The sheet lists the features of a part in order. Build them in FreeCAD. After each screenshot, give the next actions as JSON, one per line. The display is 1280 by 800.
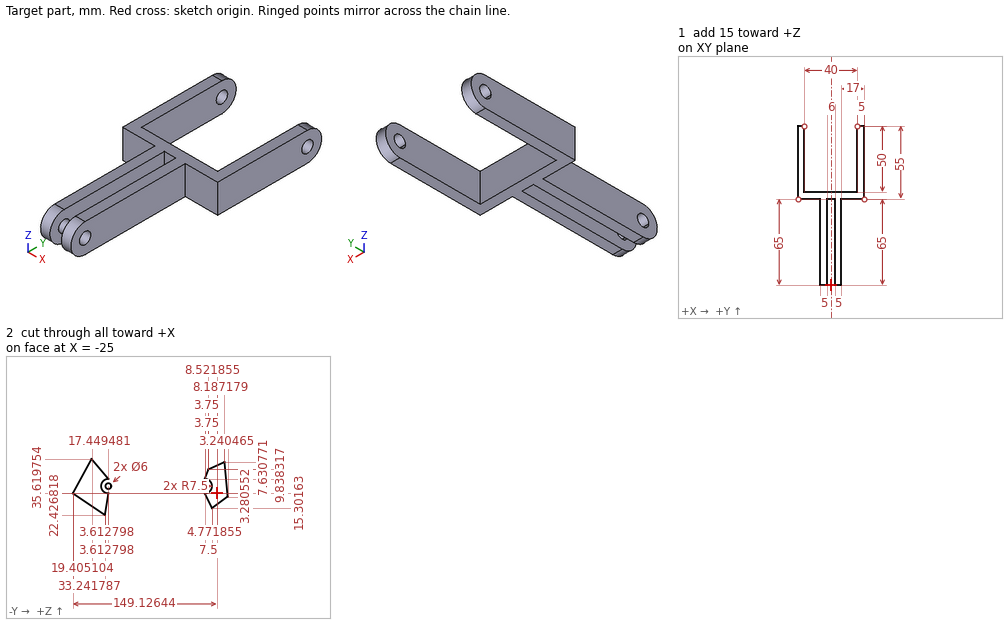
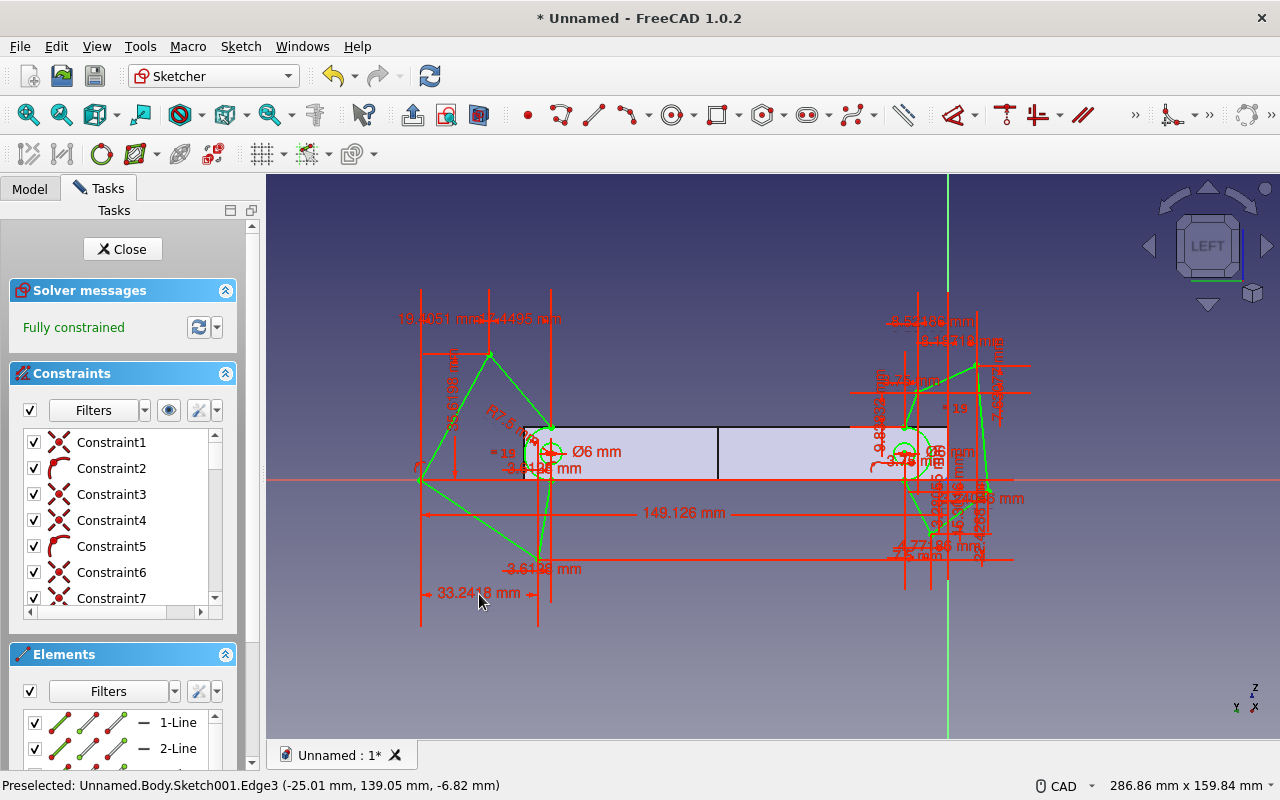
{"action": "left_click", "coordinate": [123, 249]}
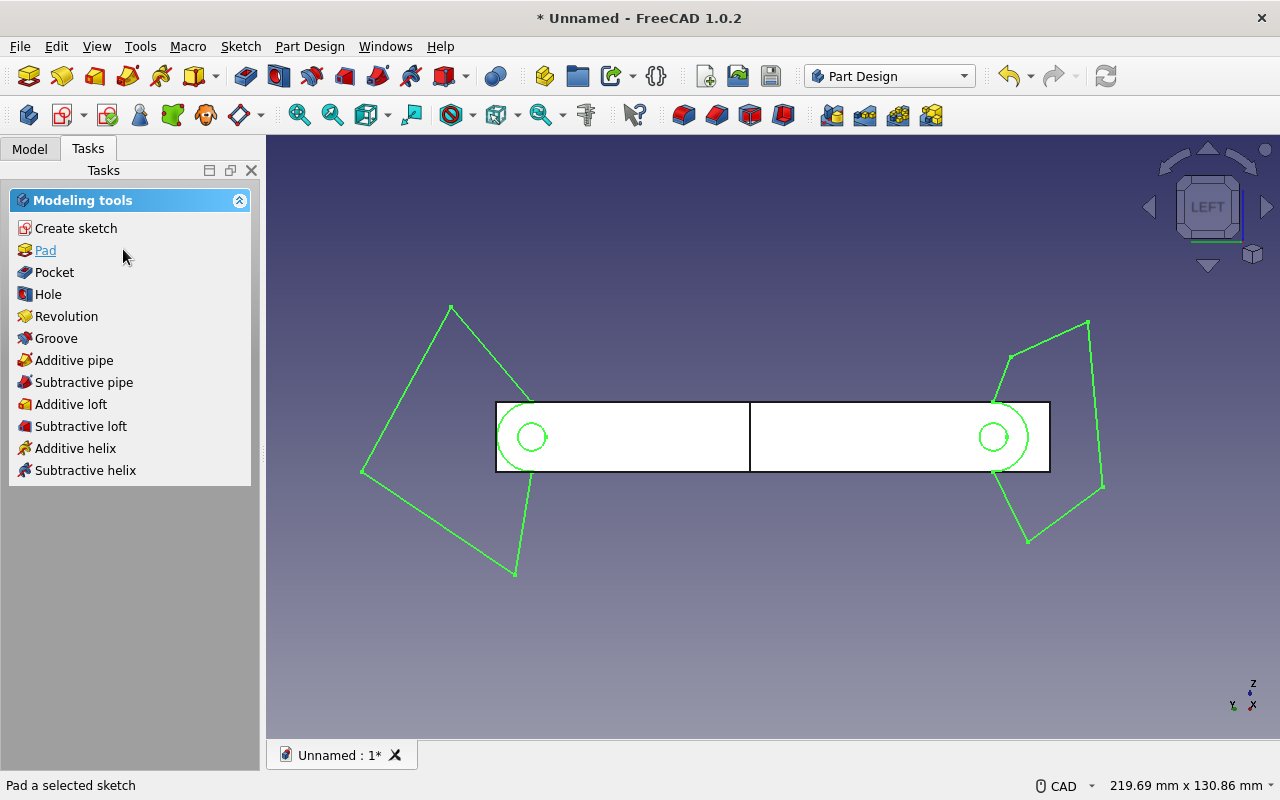
{"action": "left_click", "coordinate": [246, 76]}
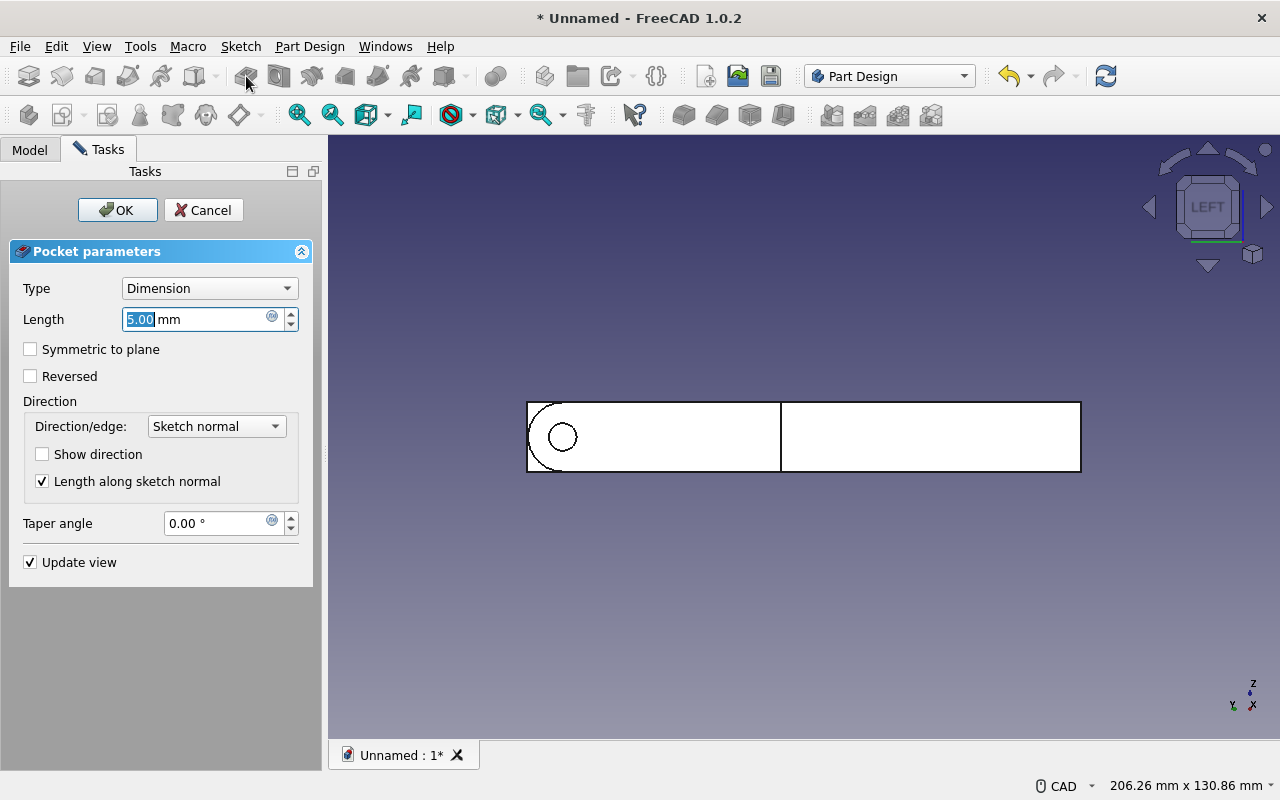
{"action": "left_click", "coordinate": [210, 288]}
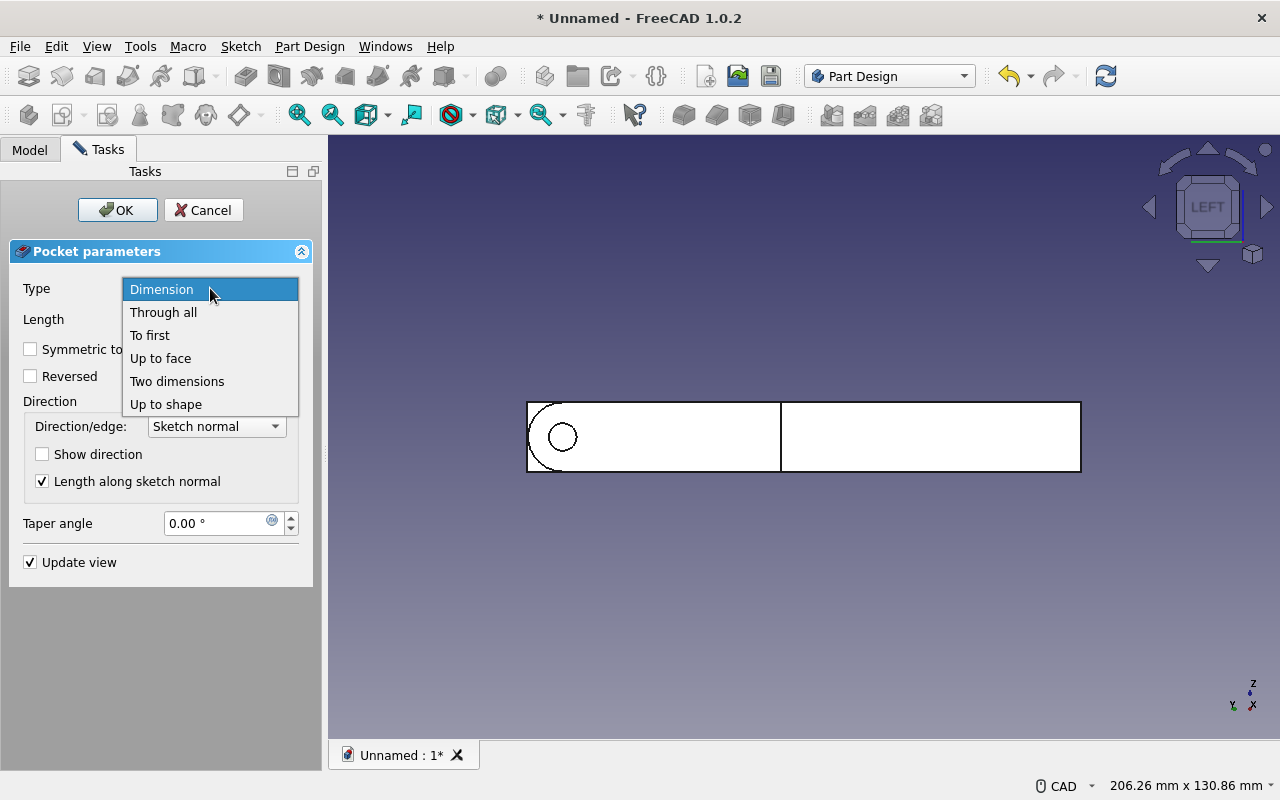
{"action": "left_click", "coordinate": [208, 312]}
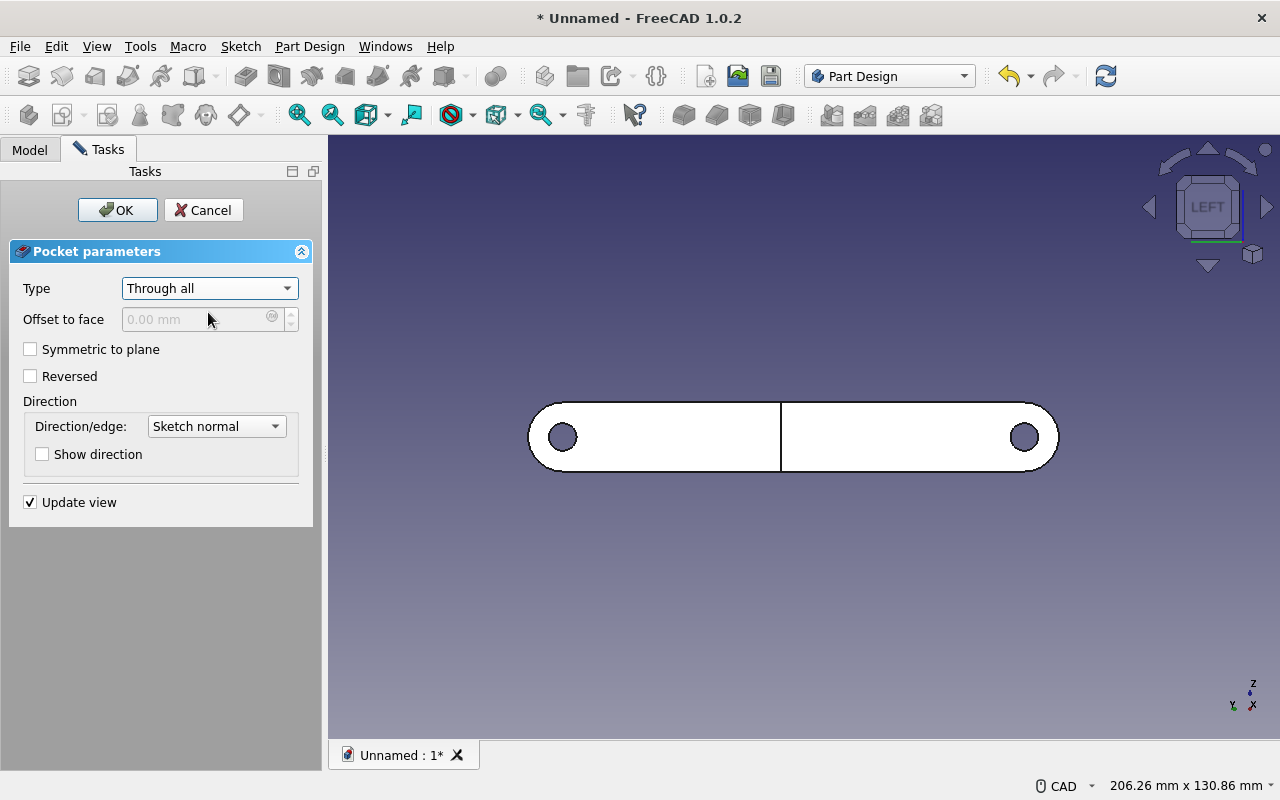
{"action": "left_click", "coordinate": [118, 210]}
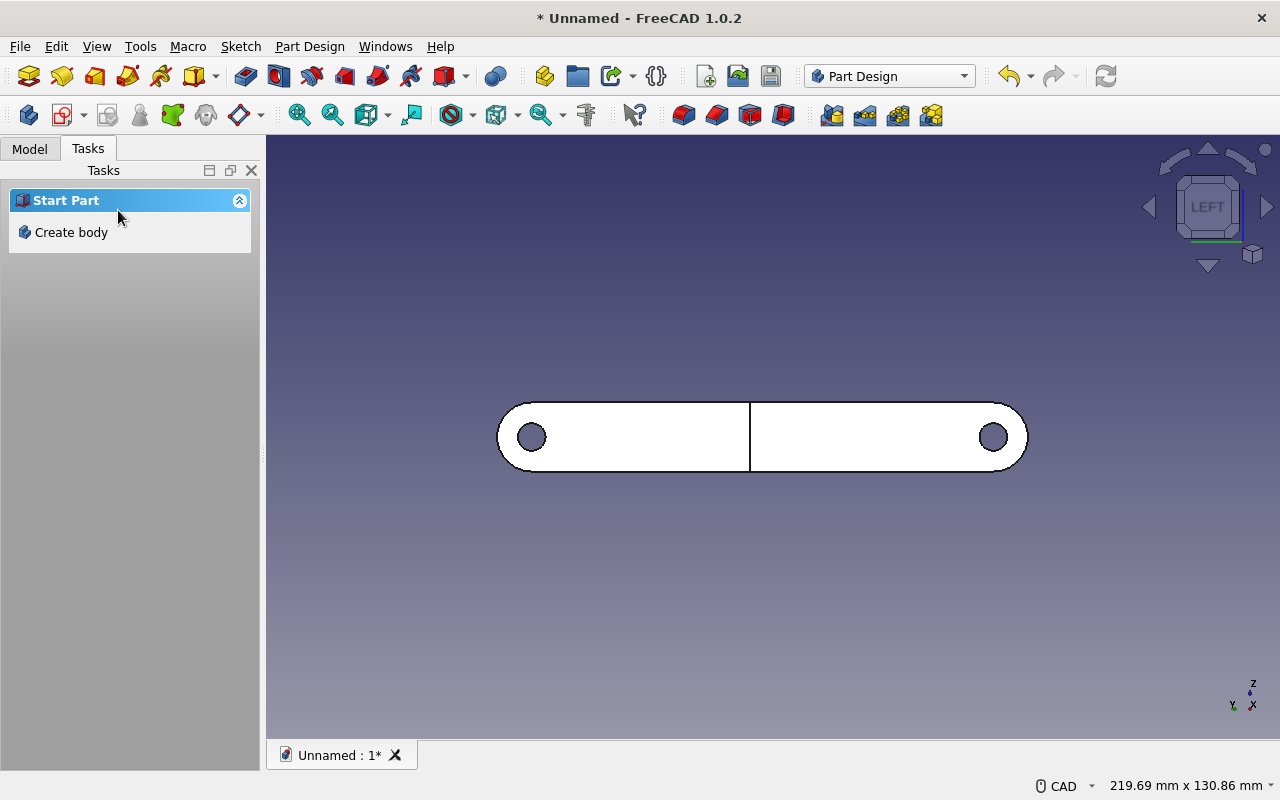
{"action": "key", "text": "0"}